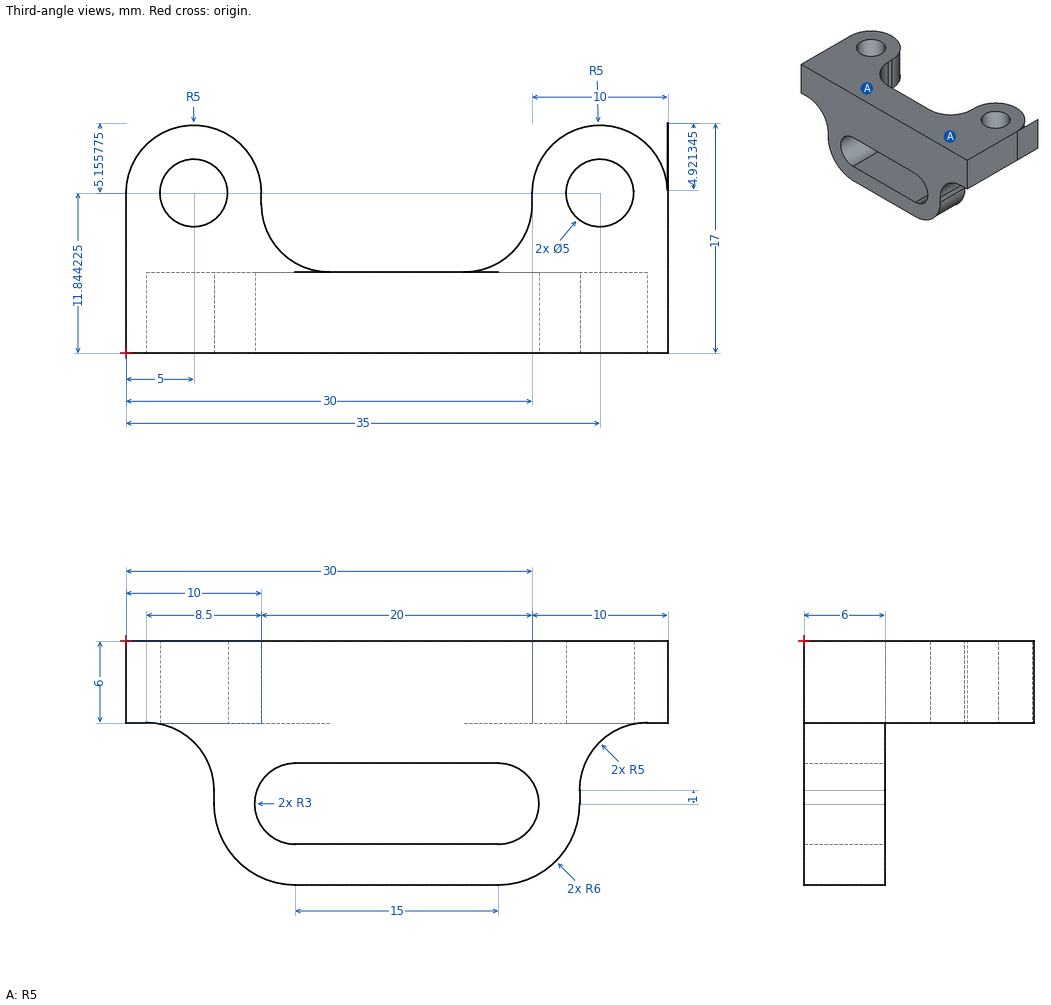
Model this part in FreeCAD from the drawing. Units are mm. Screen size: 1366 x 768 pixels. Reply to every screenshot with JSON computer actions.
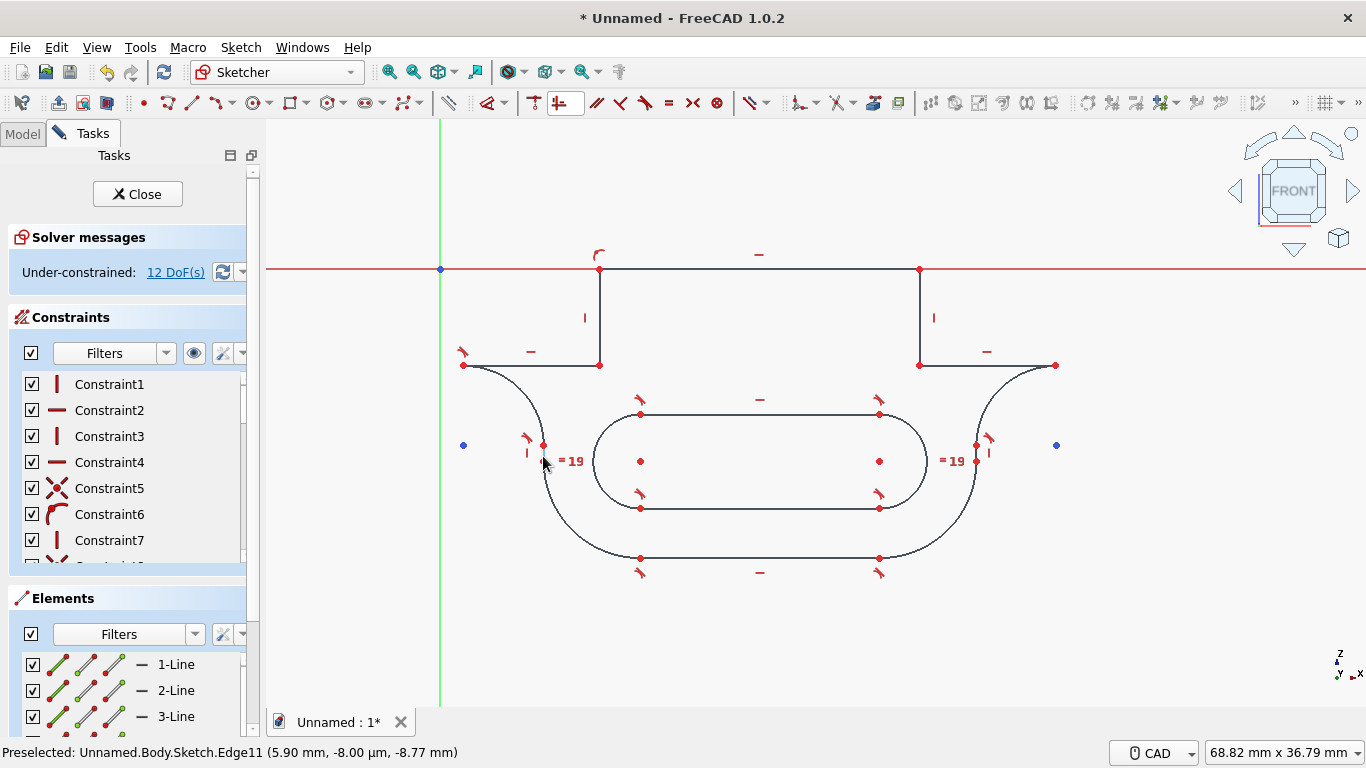
{"action": "left_click", "coordinate": [961, 366]}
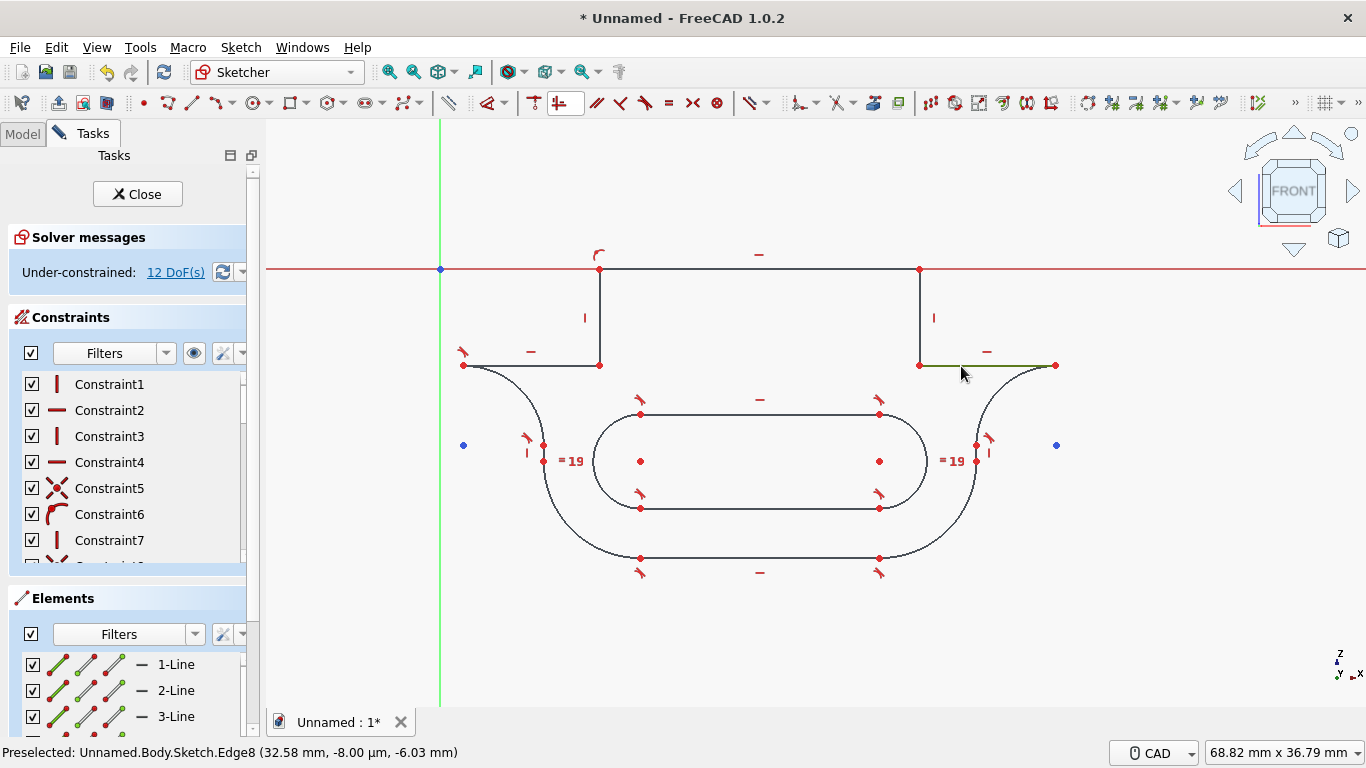
{"action": "left_click", "coordinate": [985, 410]}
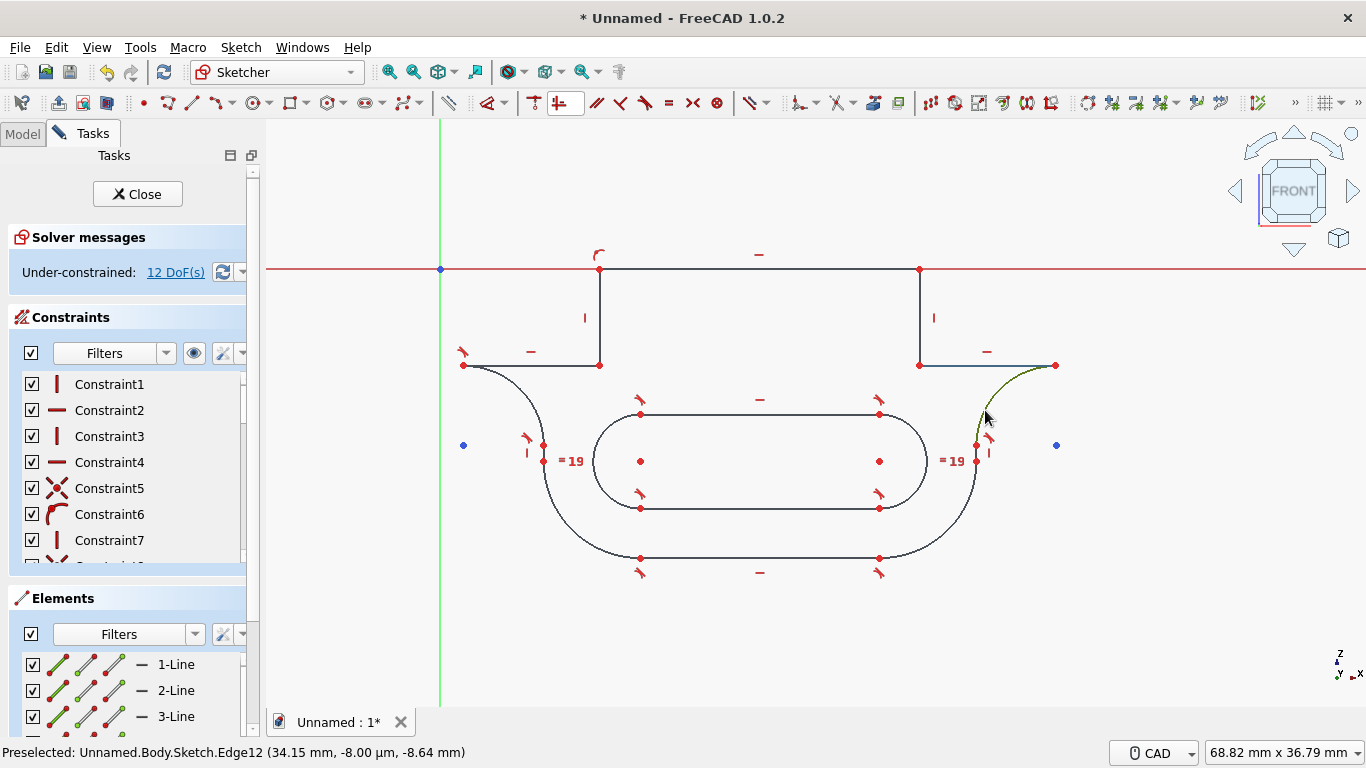
{"action": "key", "text": "t"}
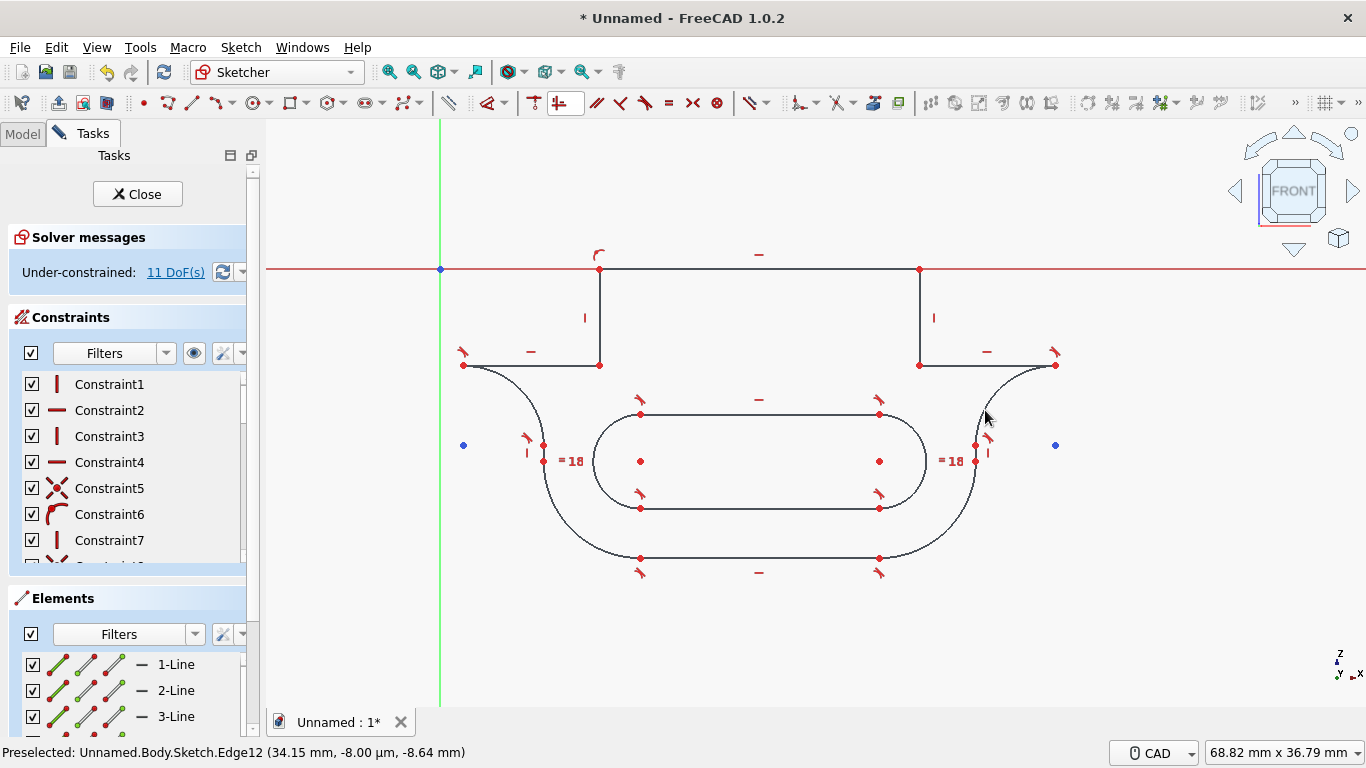
{"action": "left_click", "coordinate": [535, 410]}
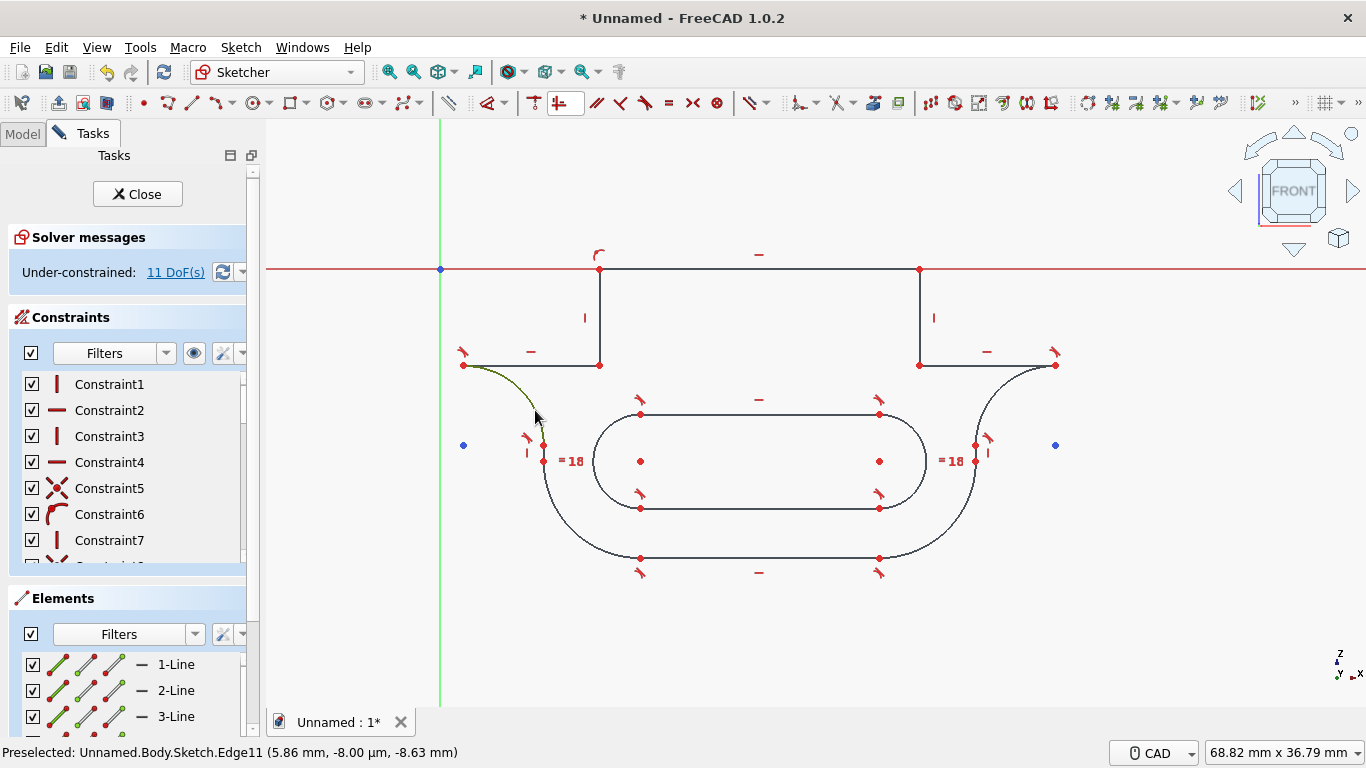
{"action": "left_click", "coordinate": [985, 410]}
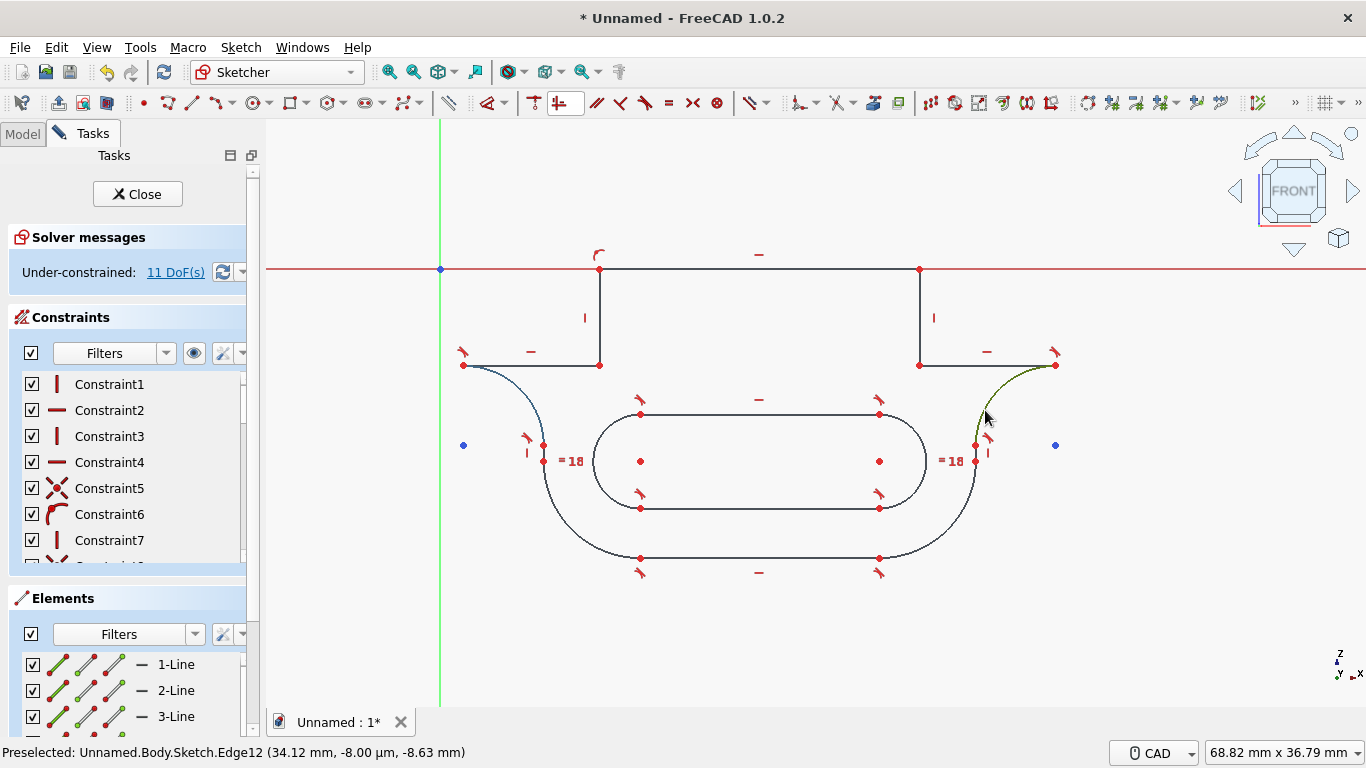
{"action": "key", "text": "e"}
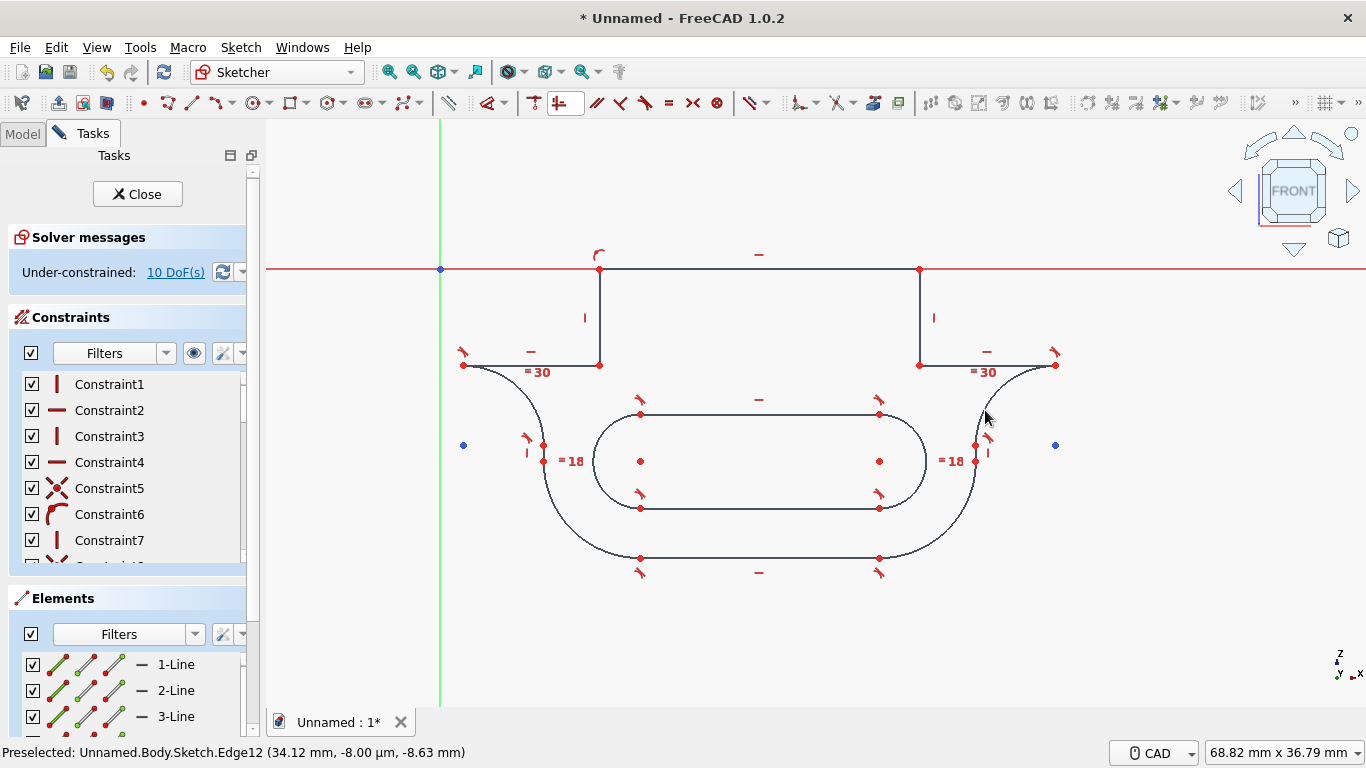
{"action": "left_click", "coordinate": [923, 548]}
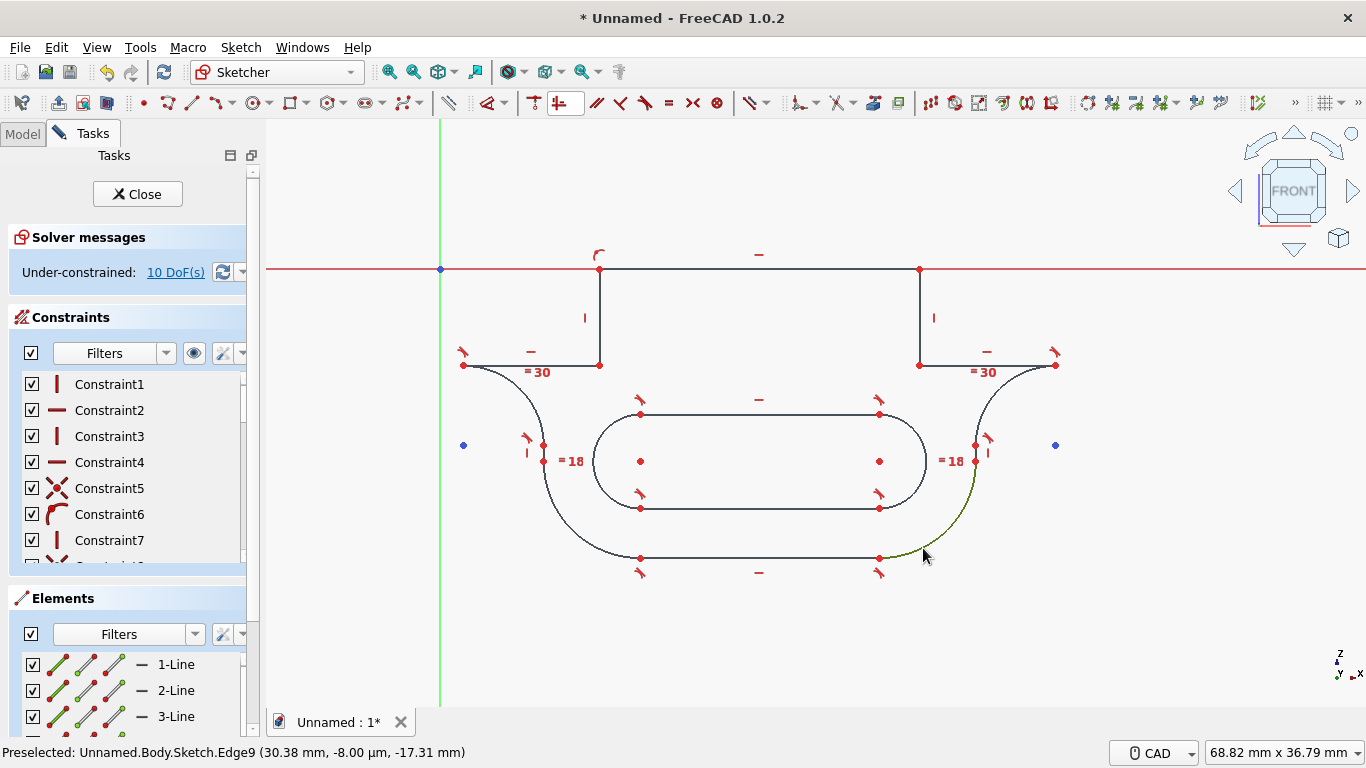
{"action": "key", "text": "k r"}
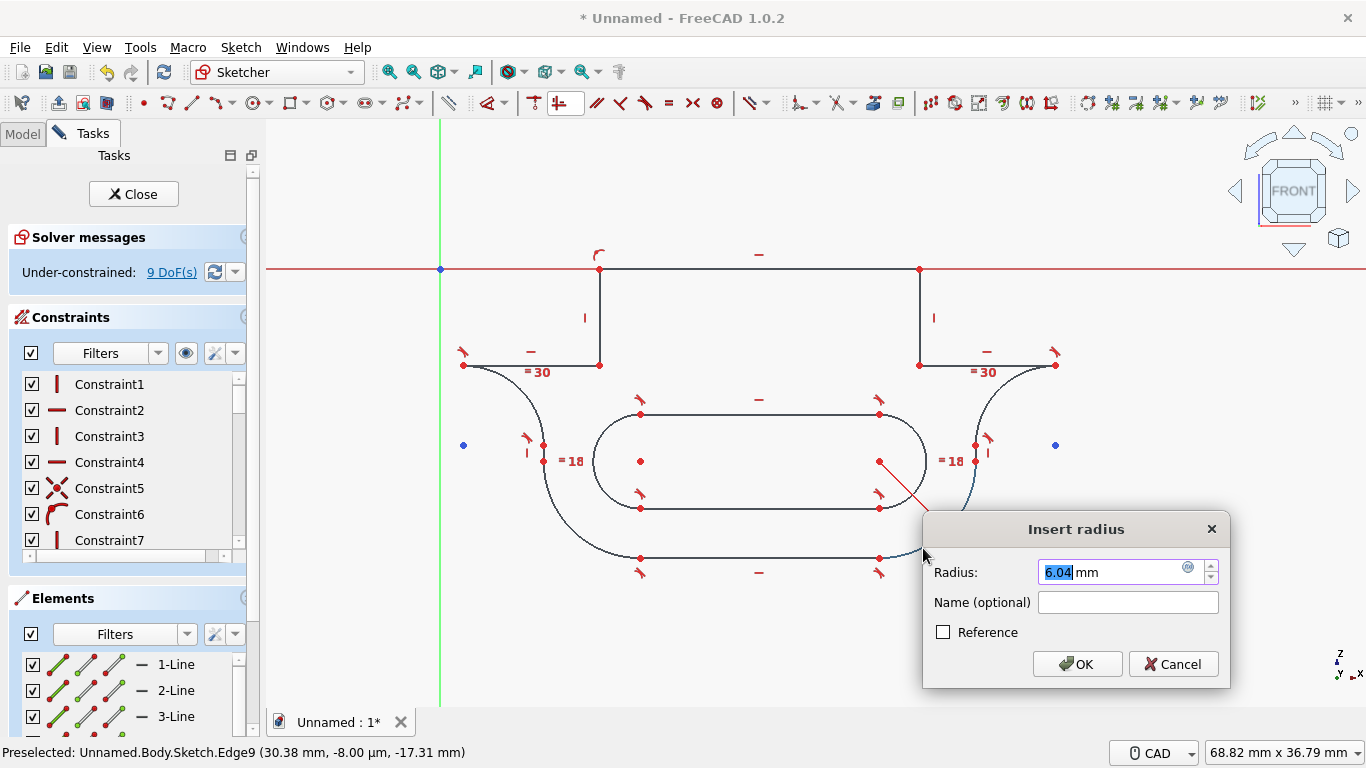
{"action": "type", "text": "6"}
{"action": "key", "text": "Return"}